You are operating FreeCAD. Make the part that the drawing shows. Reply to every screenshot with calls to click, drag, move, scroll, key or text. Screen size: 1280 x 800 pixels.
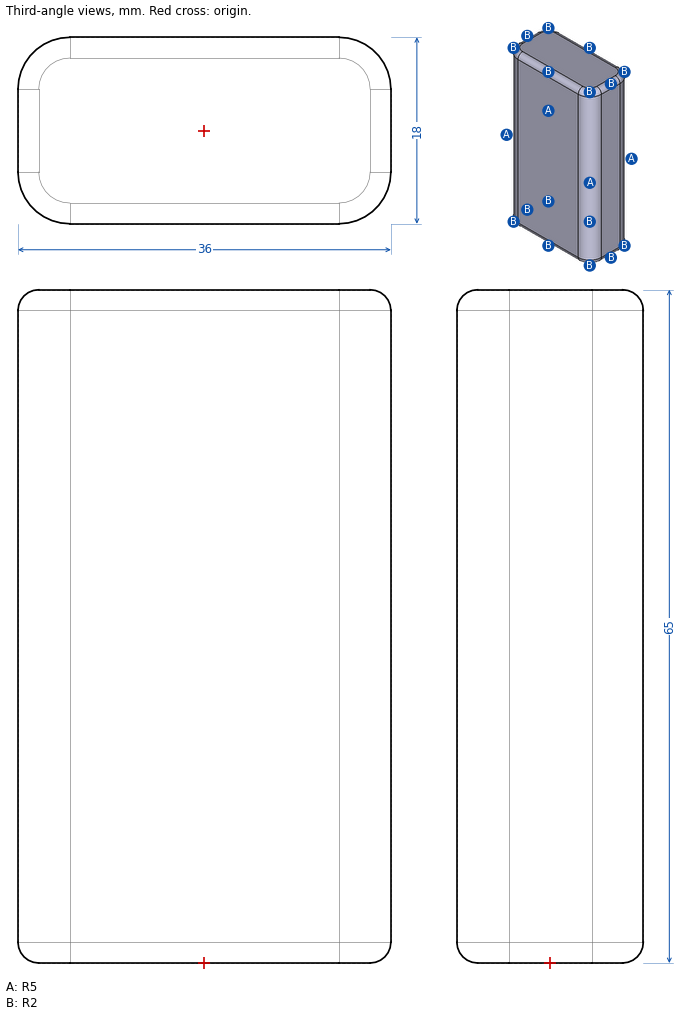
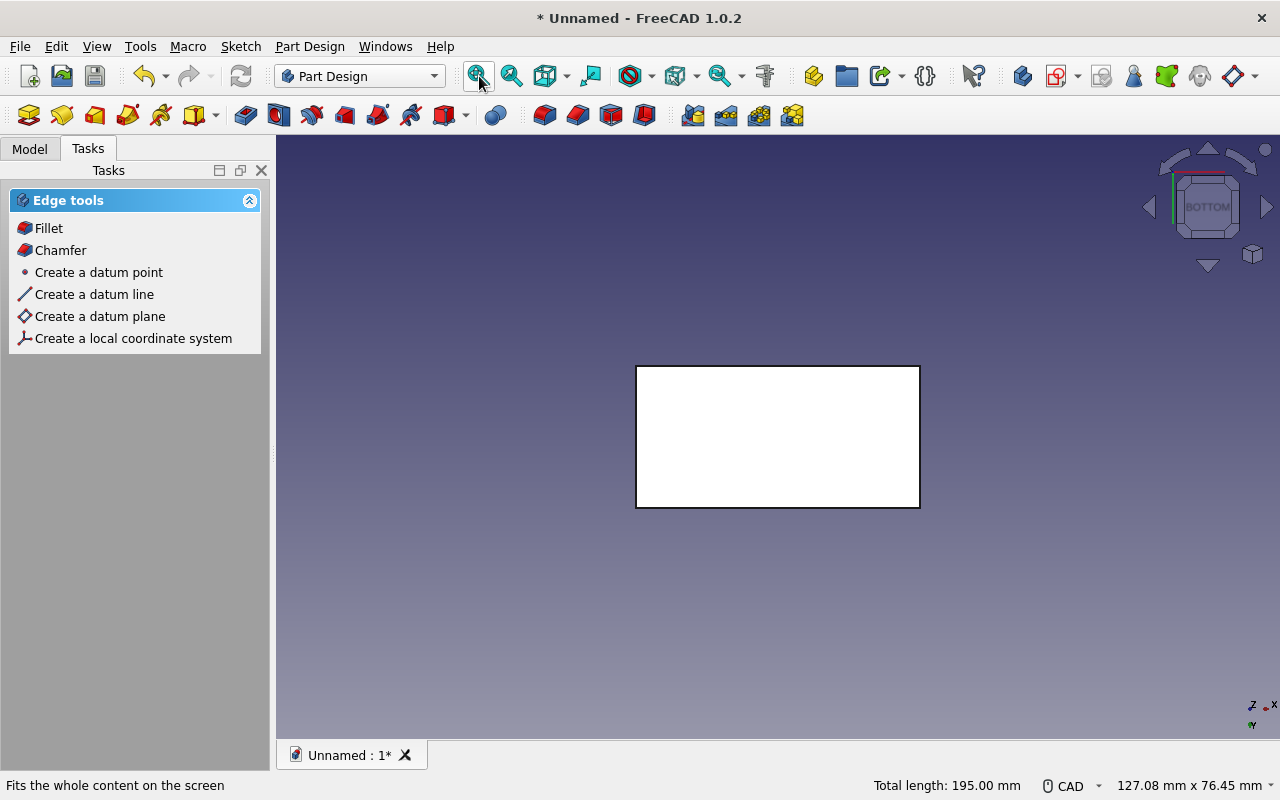
key(4)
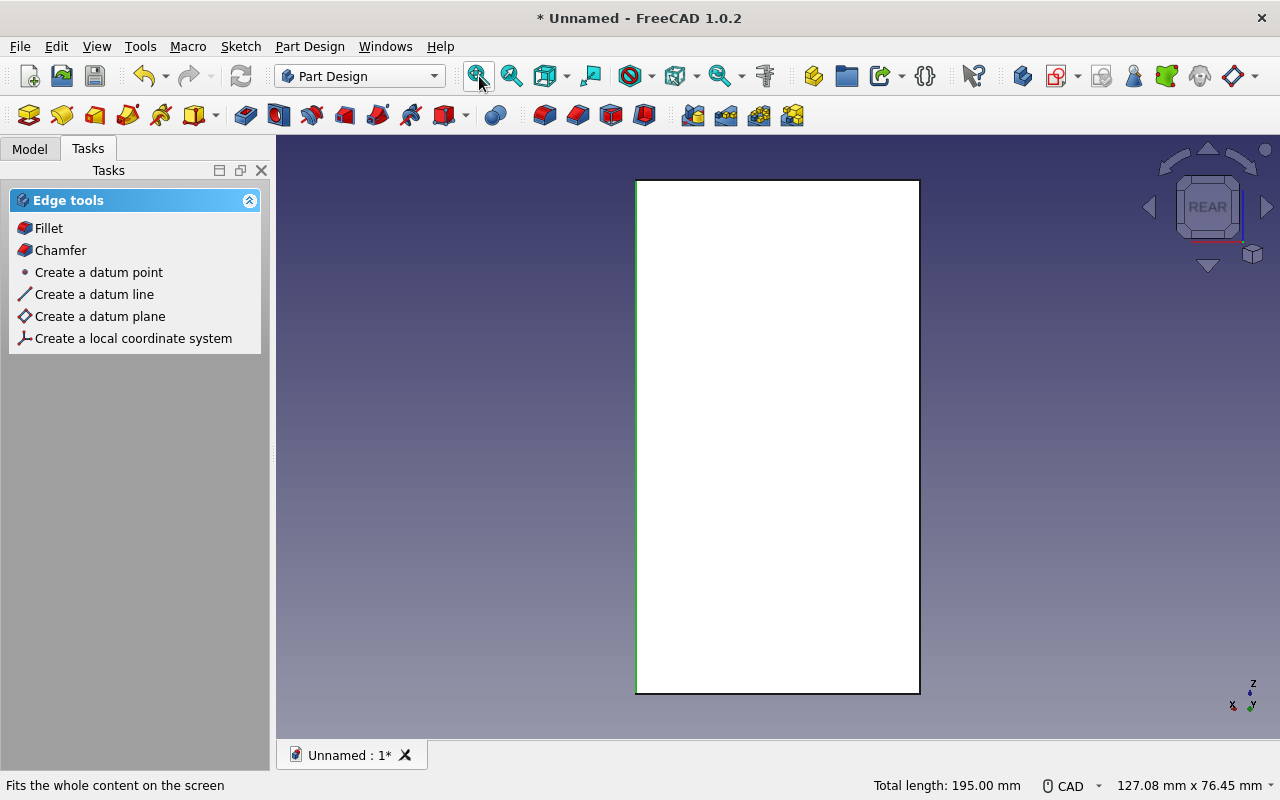
click(920, 436, ctrl)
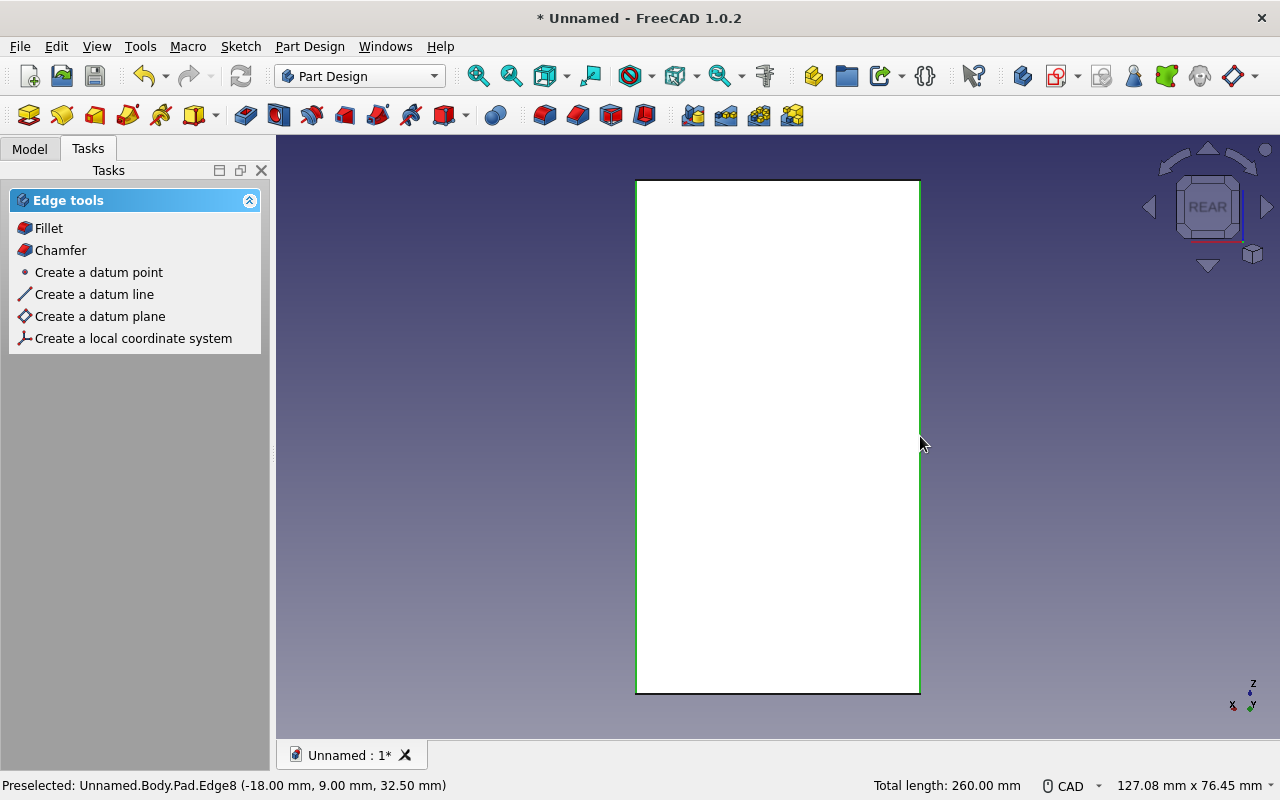
click(545, 116)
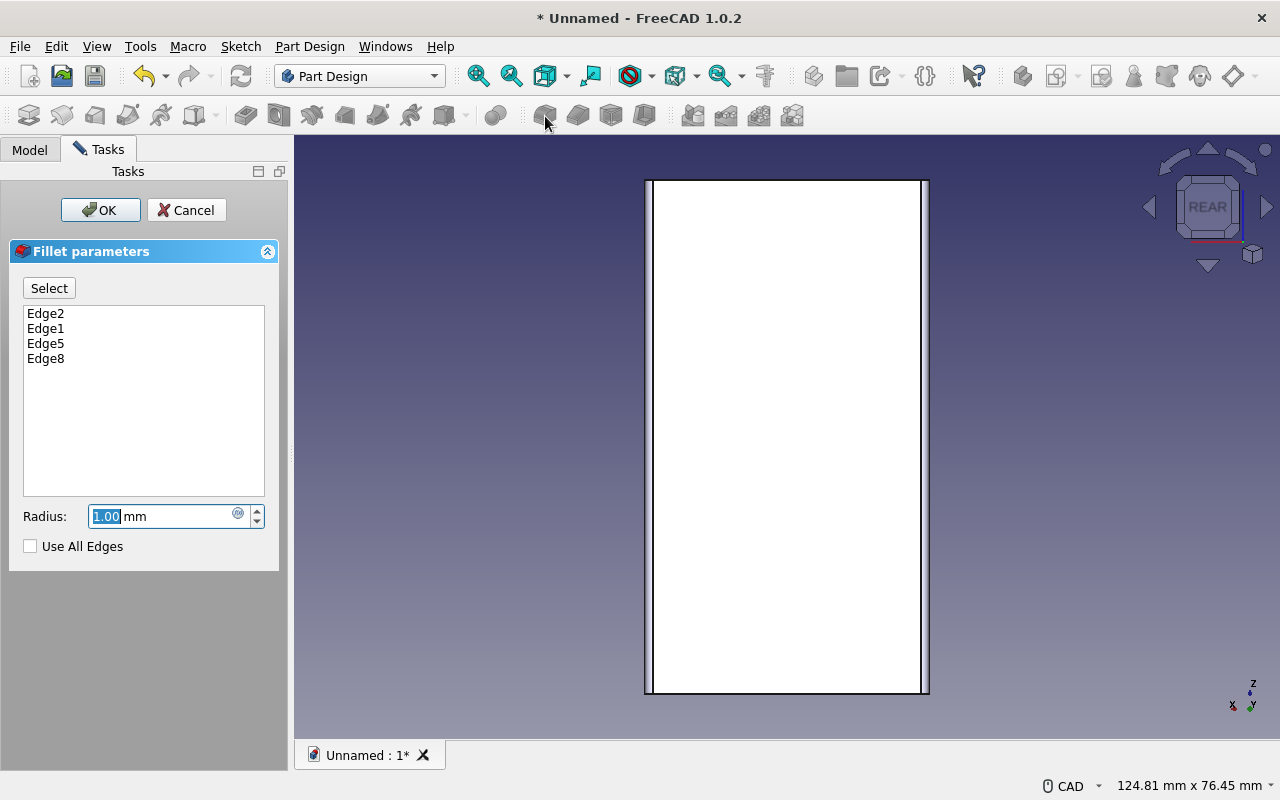
text(5)
key(Tab)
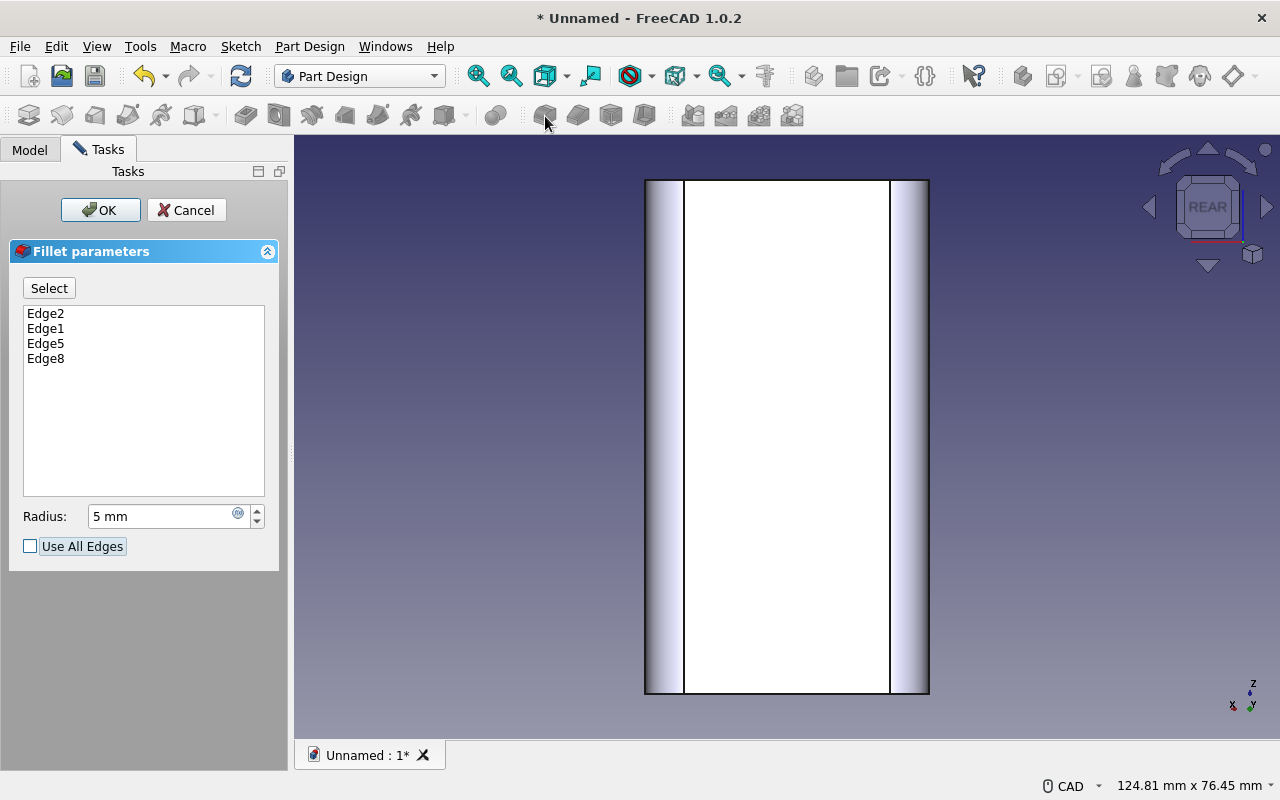
click(101, 210)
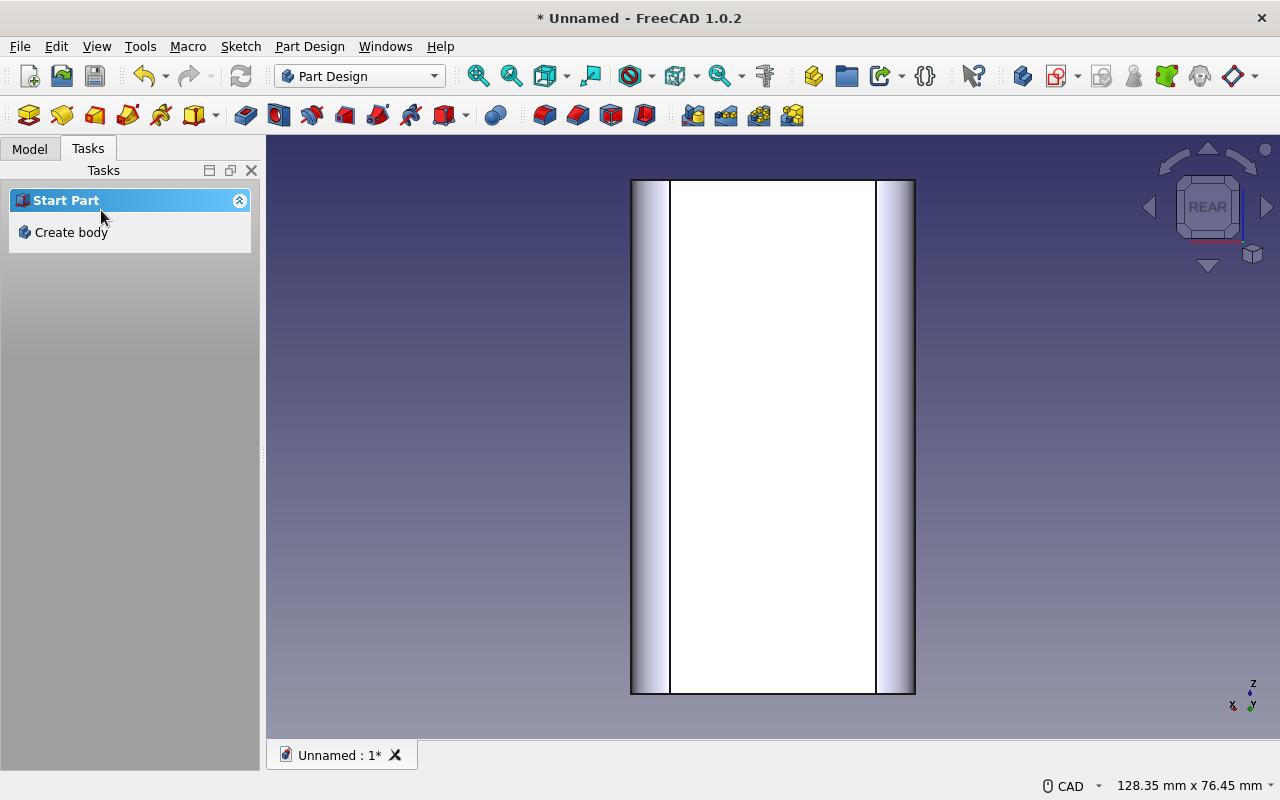
key(0)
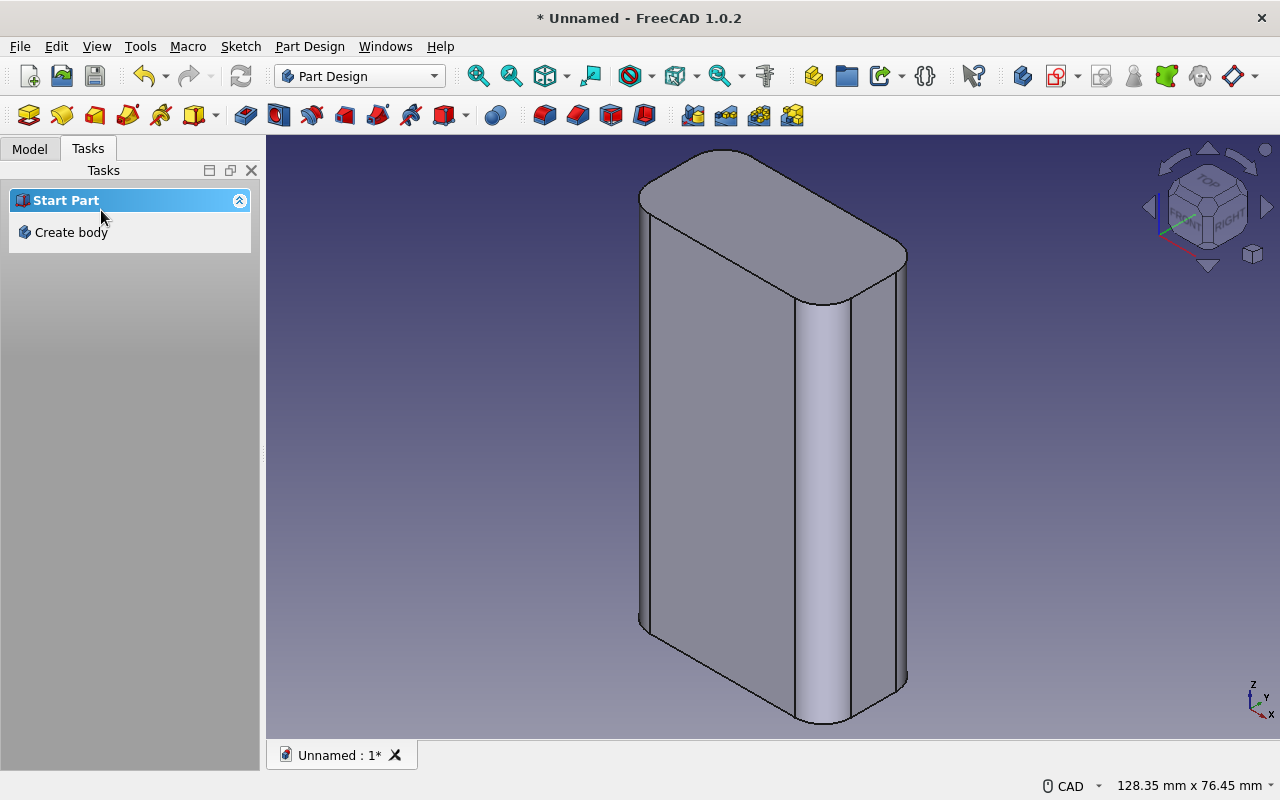
click(802, 243)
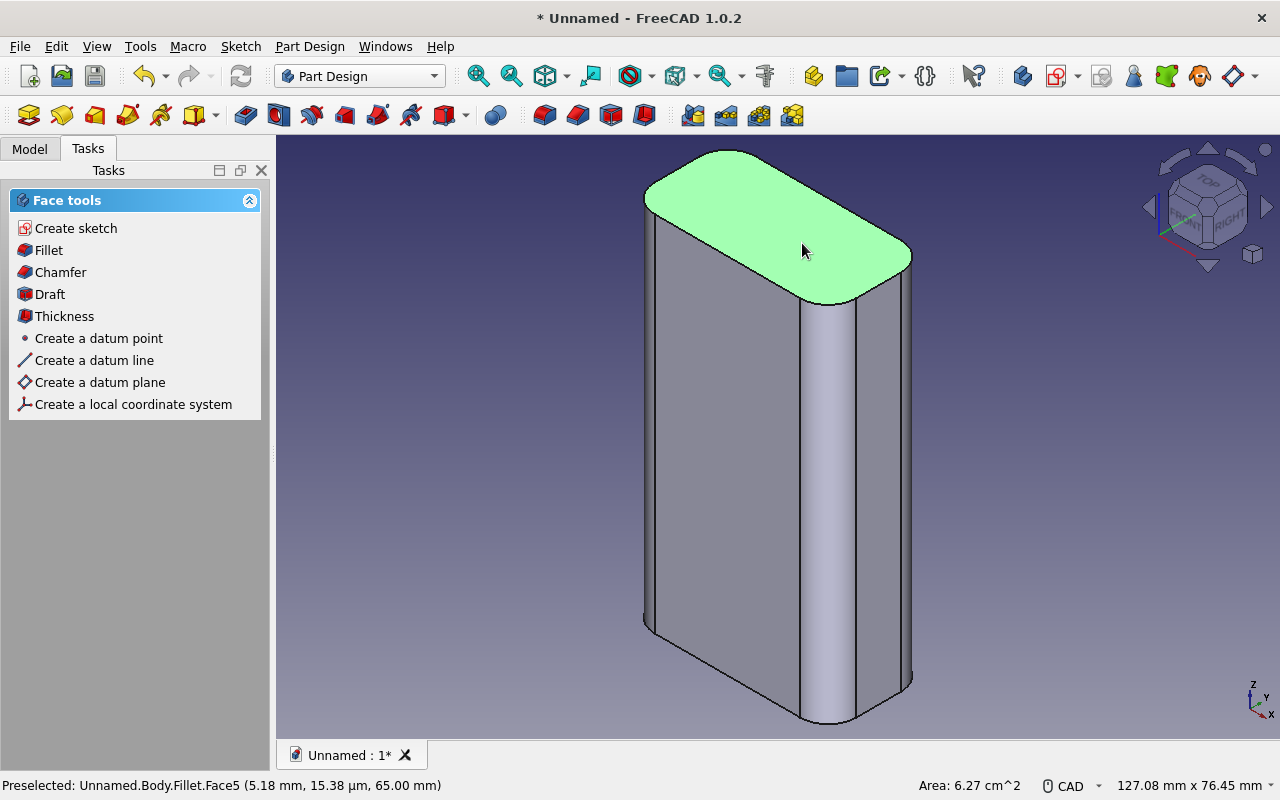
key(2)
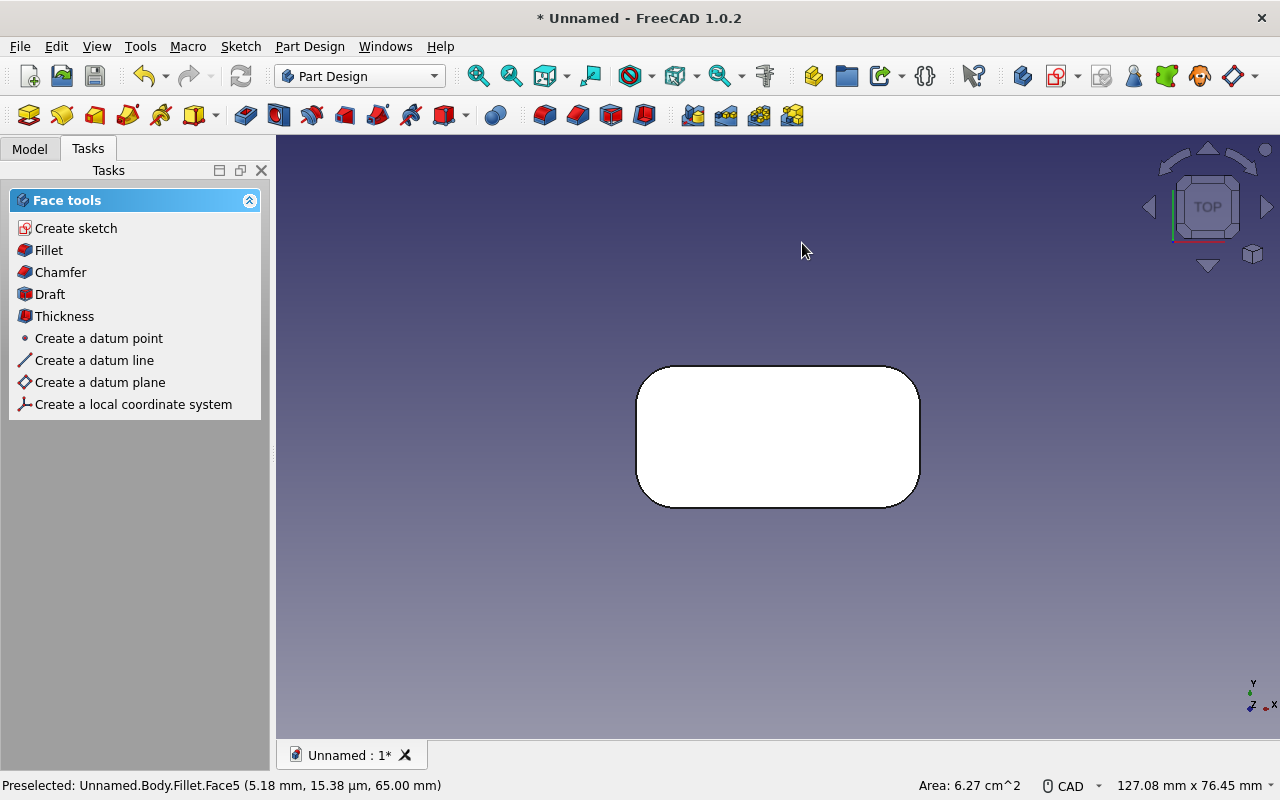
click(479, 76)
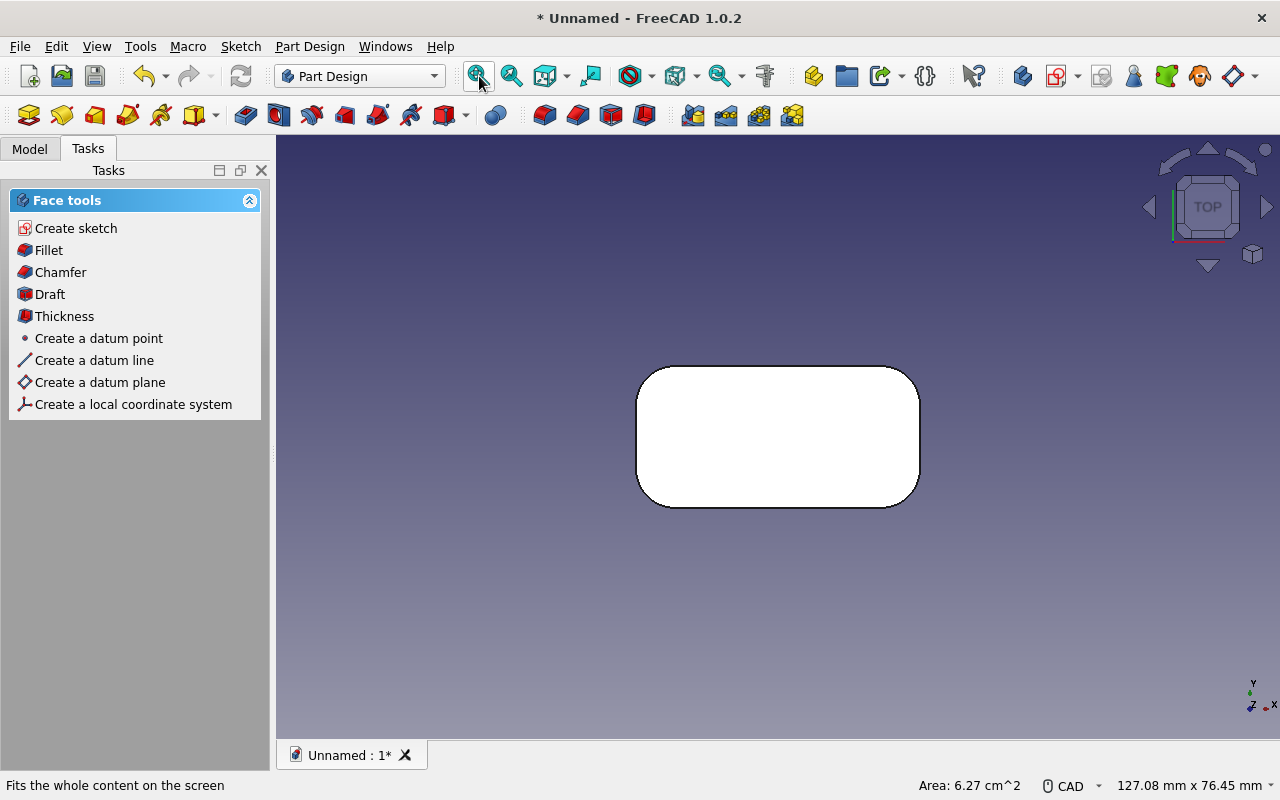
key(1)